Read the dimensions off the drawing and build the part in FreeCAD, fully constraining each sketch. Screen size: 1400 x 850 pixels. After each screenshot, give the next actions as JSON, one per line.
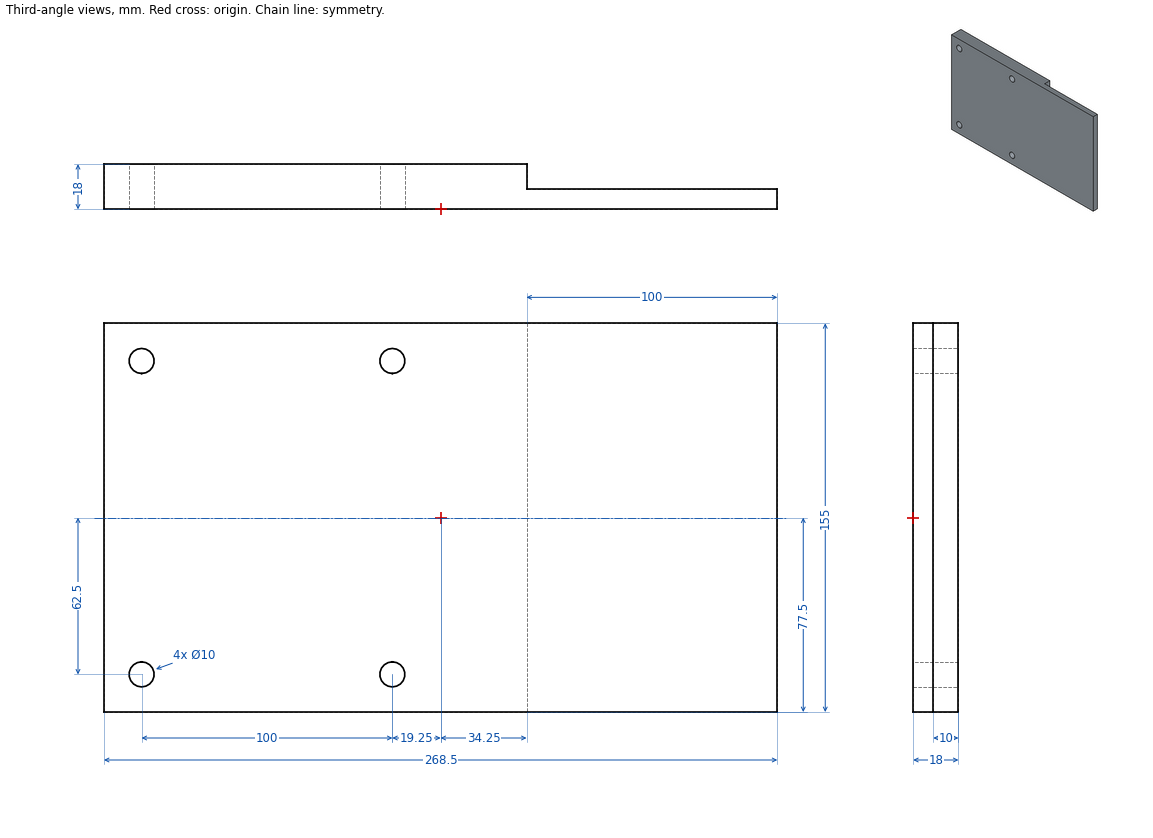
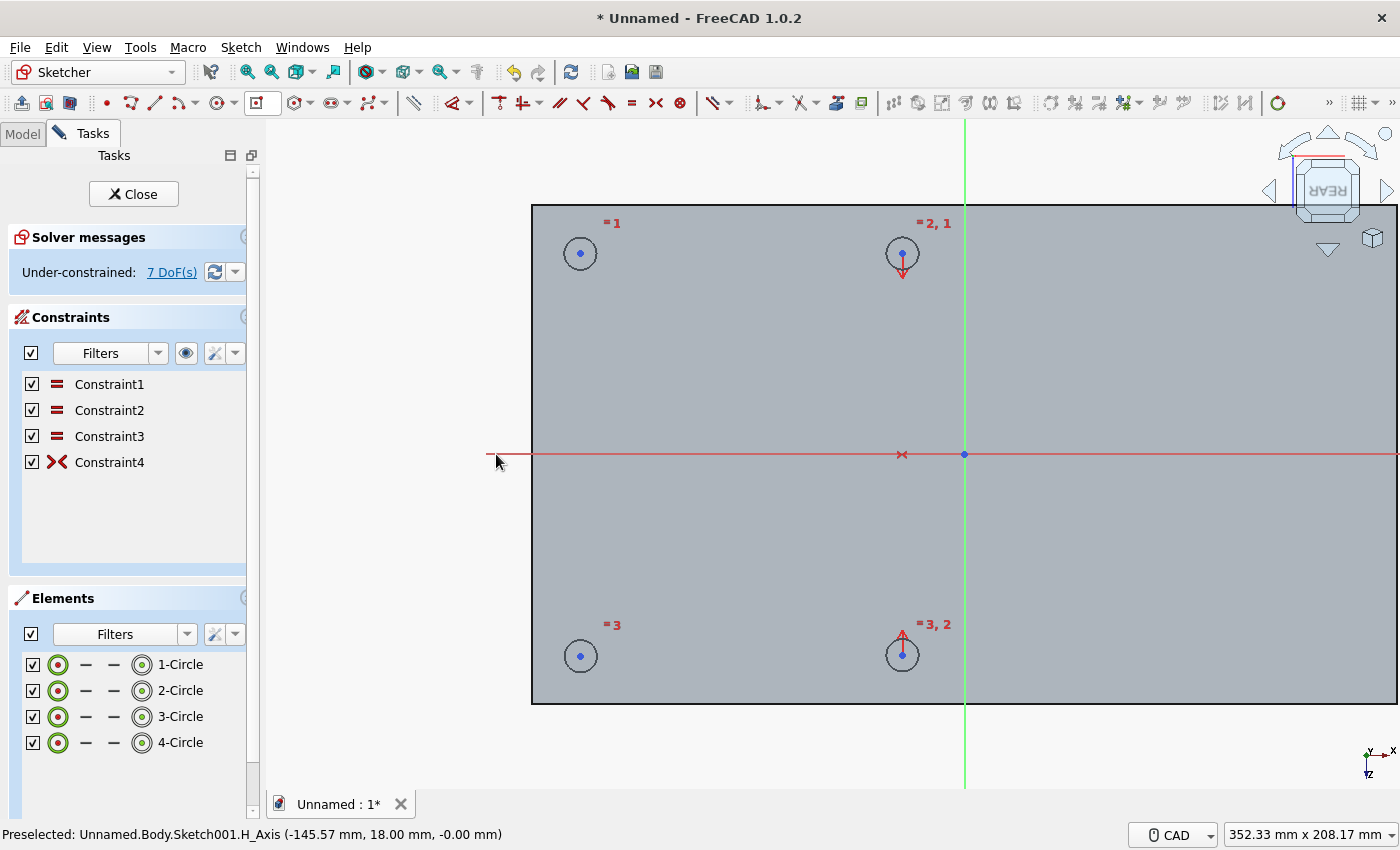
{"action": "left_click", "coordinate": [580, 254]}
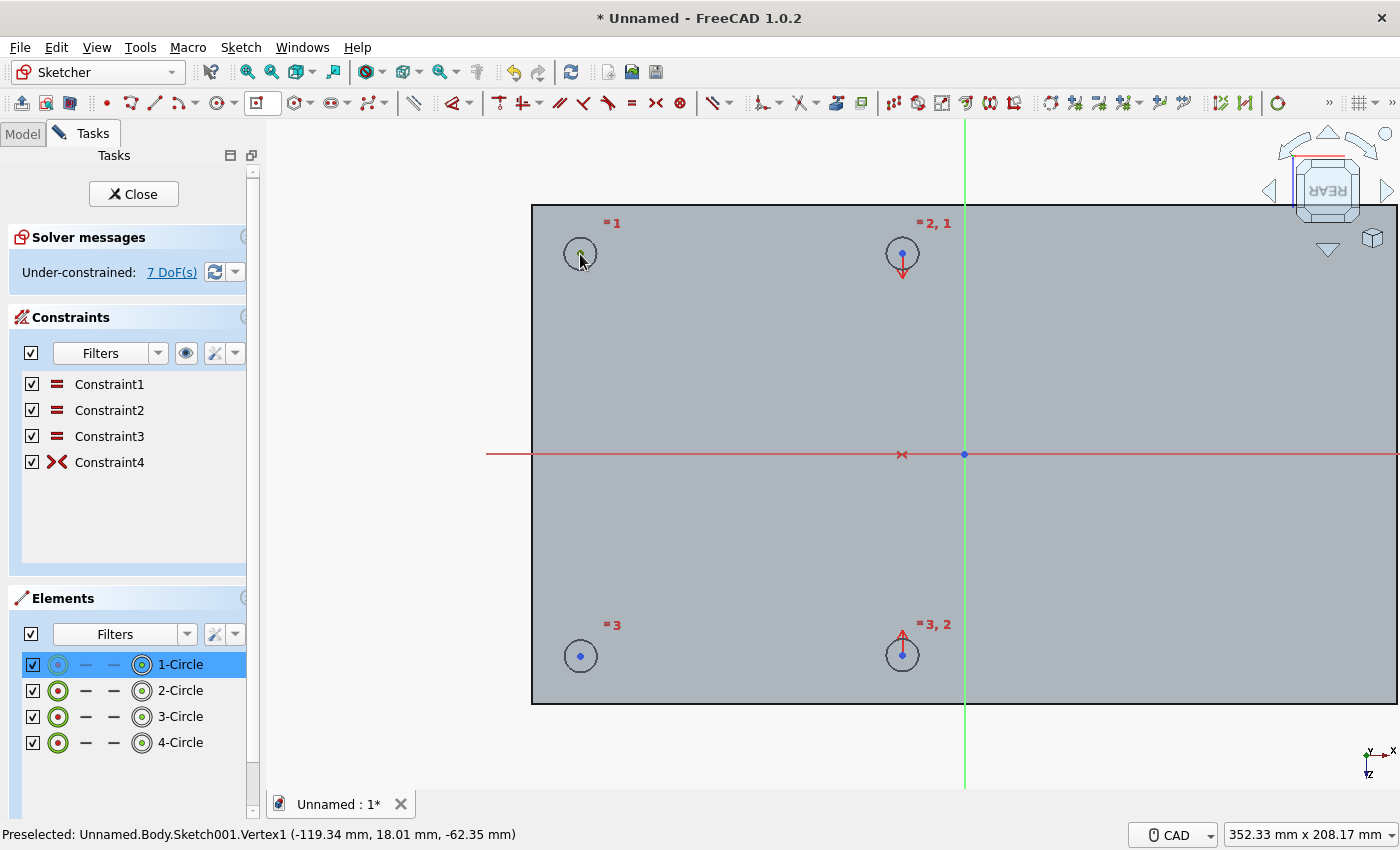
{"action": "left_click", "coordinate": [581, 656]}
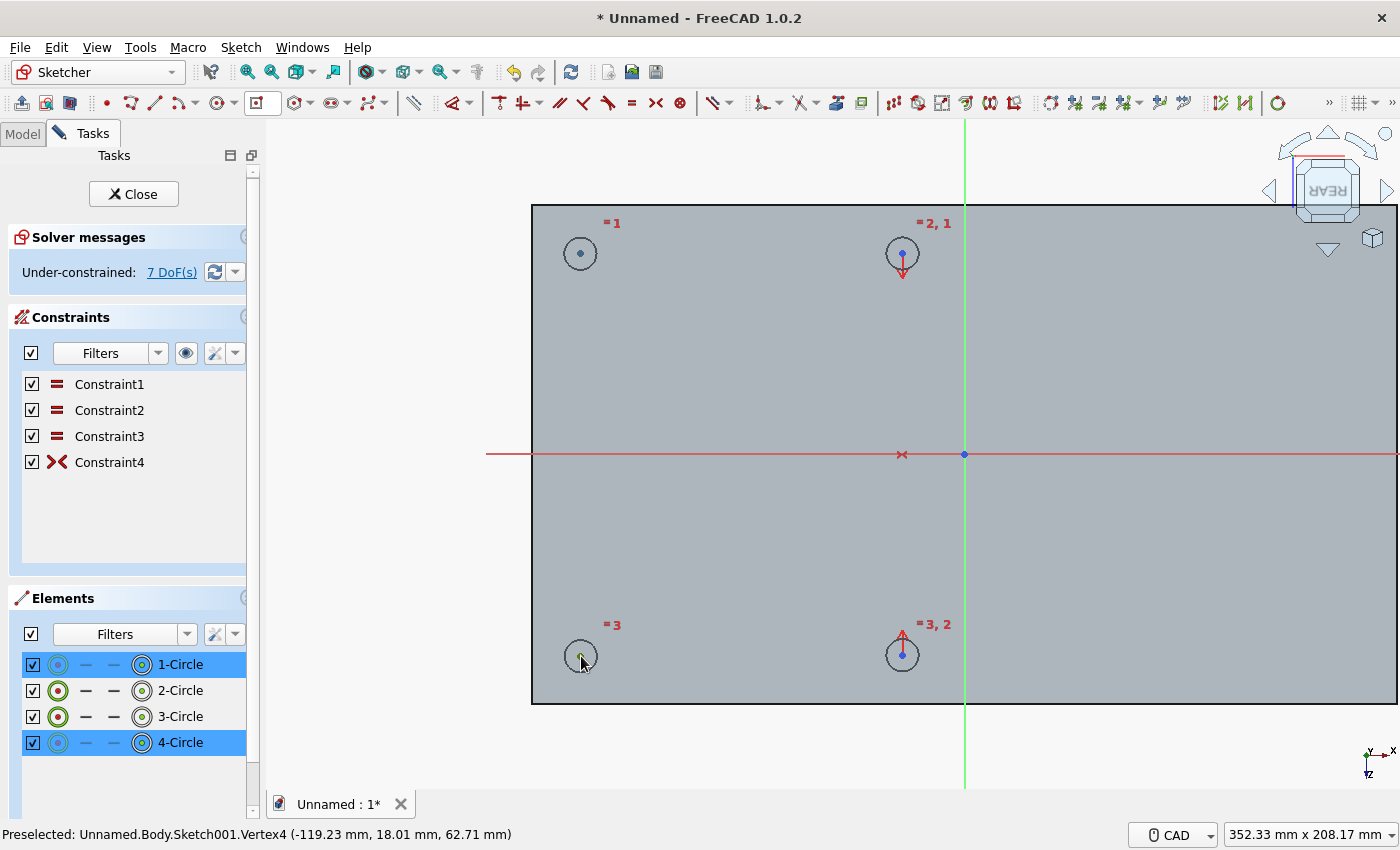
{"action": "left_click", "coordinate": [496, 454]}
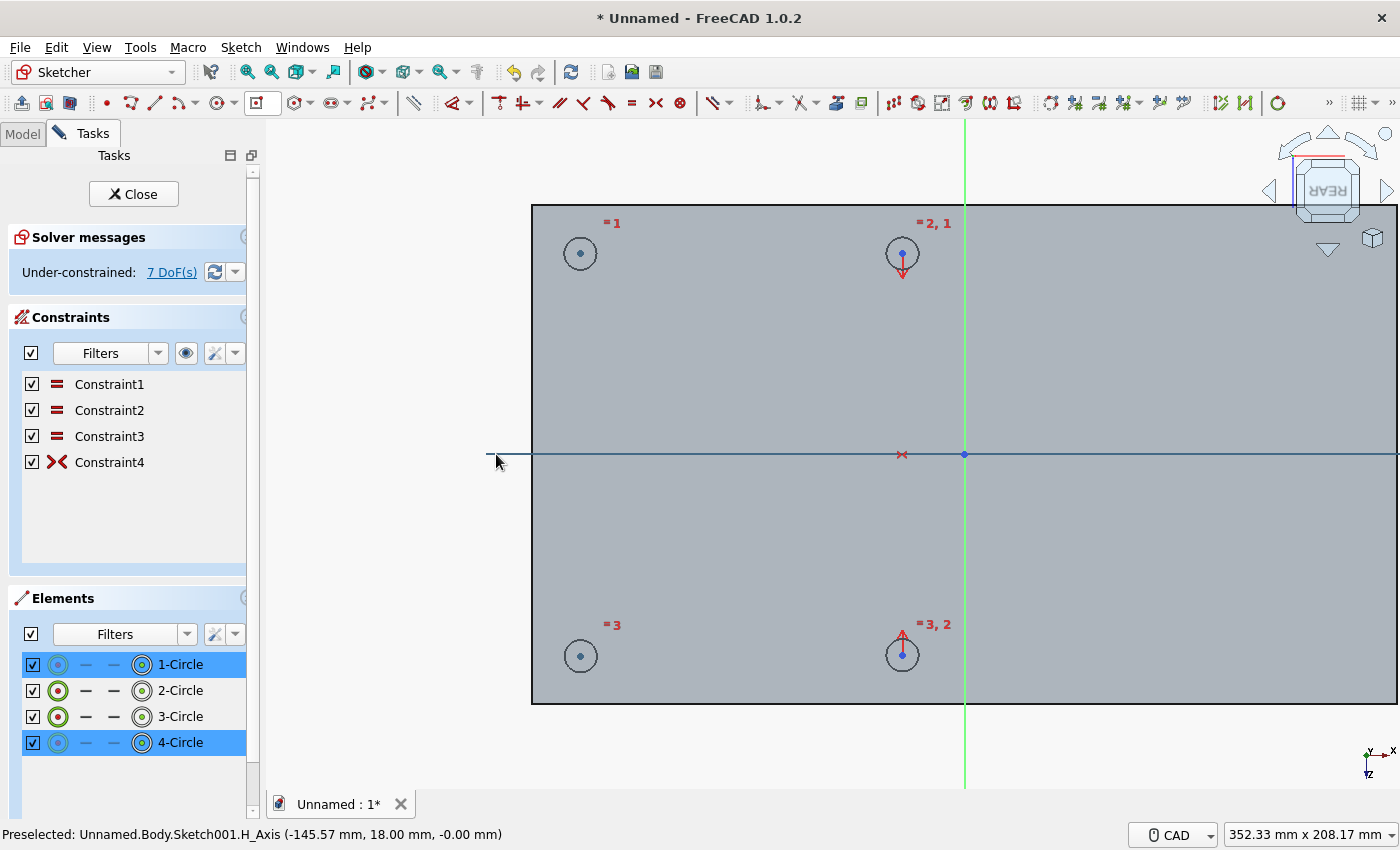
{"action": "left_click", "coordinate": [656, 104]}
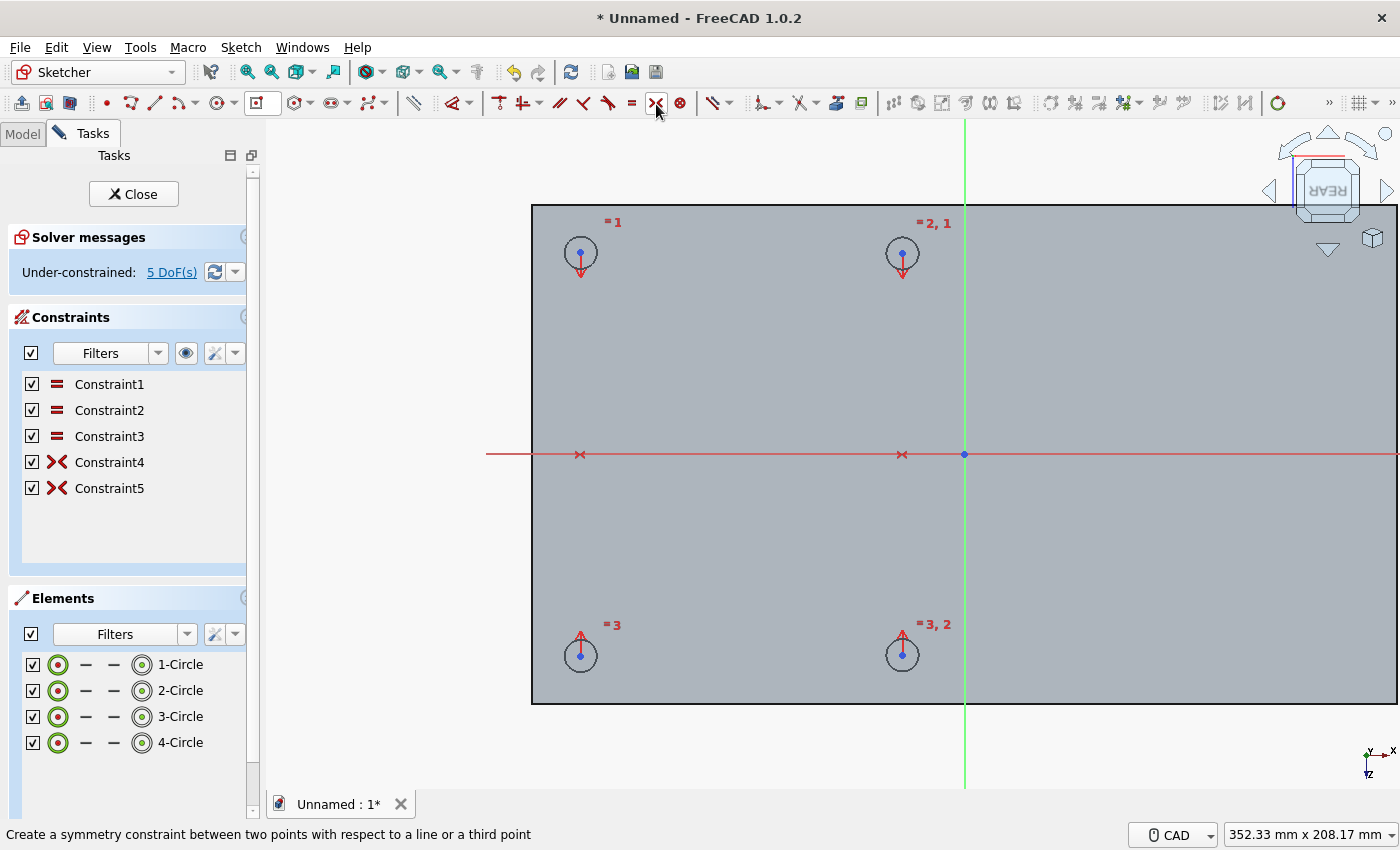
{"action": "left_click", "coordinate": [452, 104]}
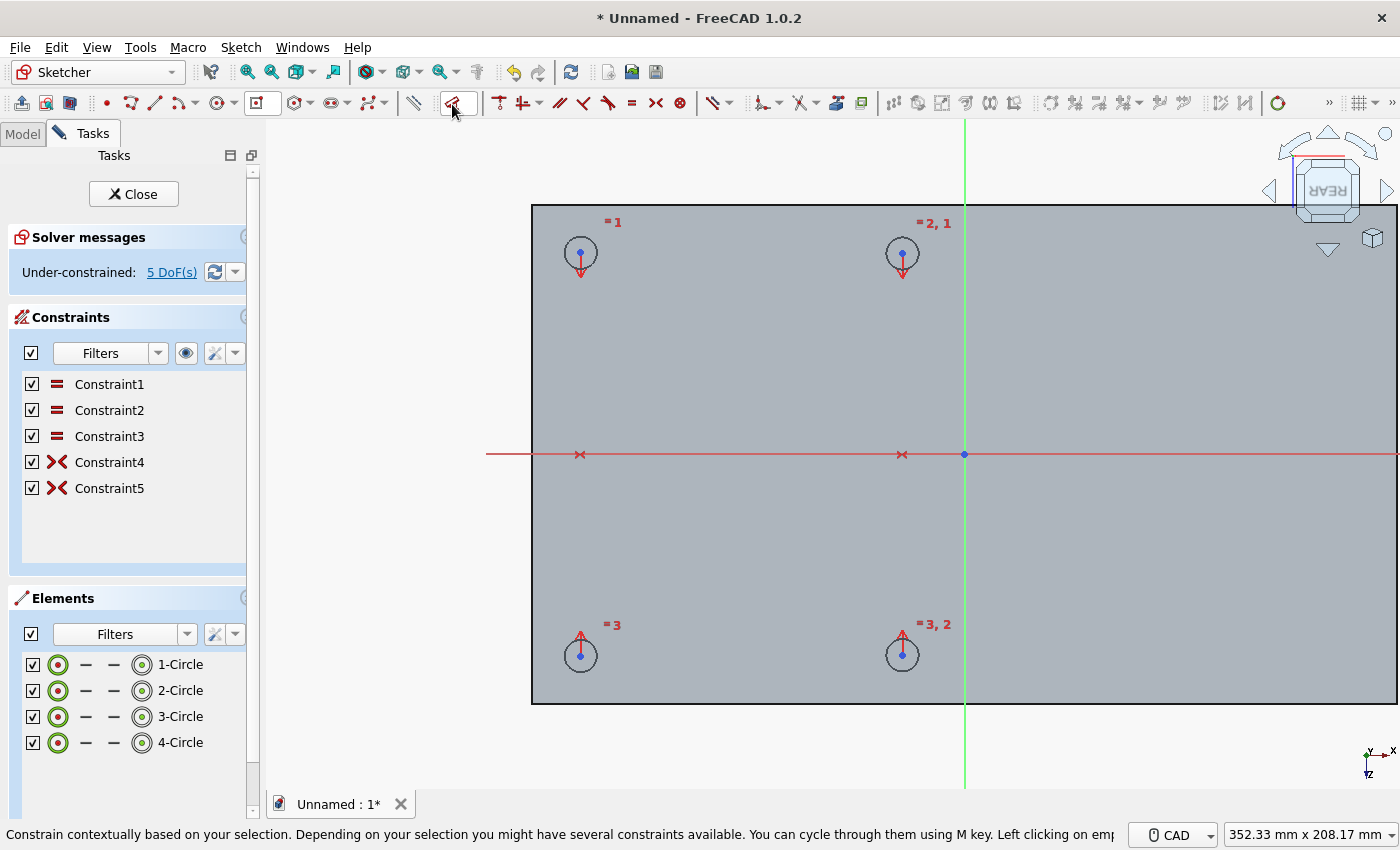
{"action": "scroll", "coordinate": [592, 241], "scroll_direction": "up", "scroll_amount": 2}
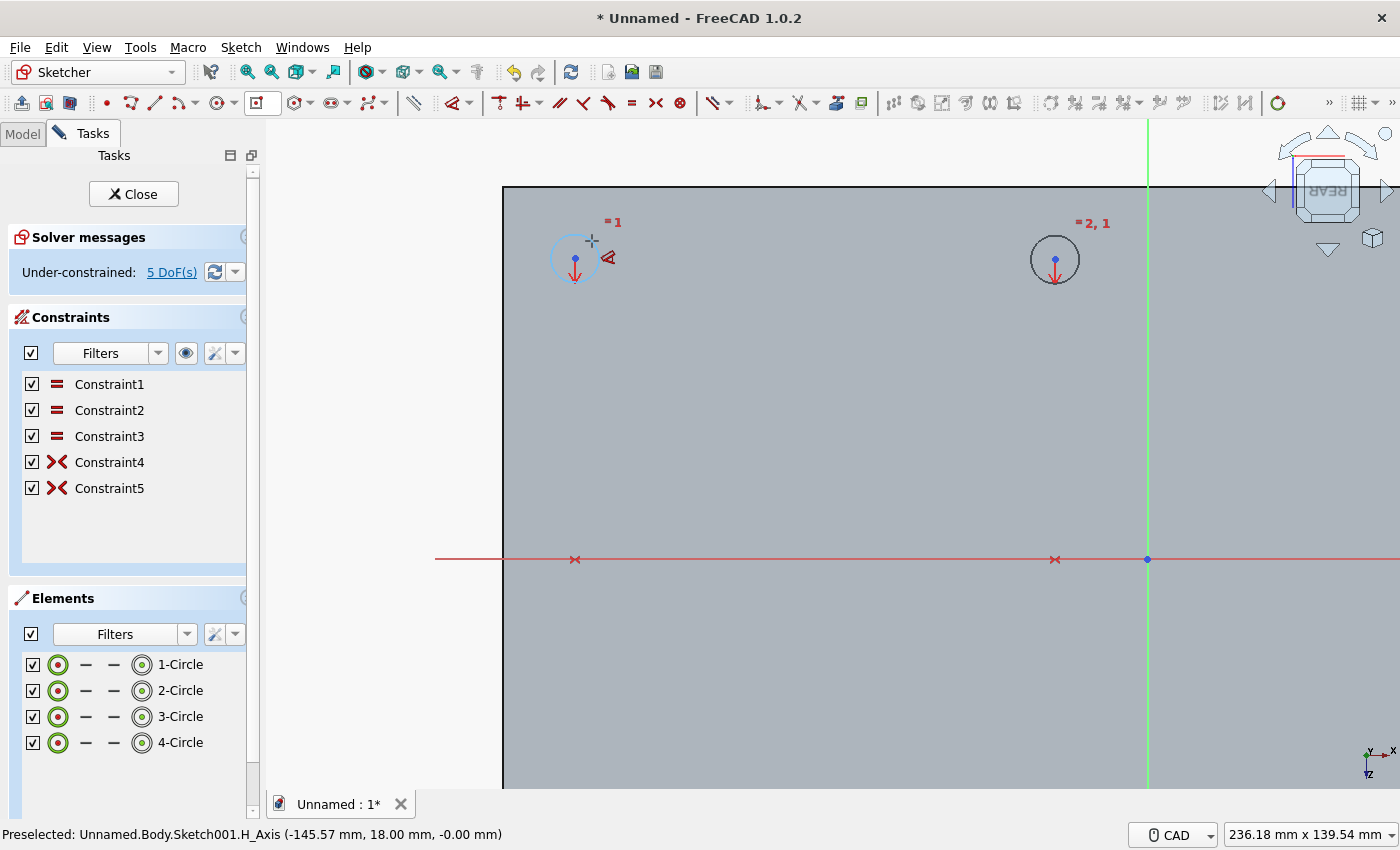
{"action": "left_click", "coordinate": [592, 241]}
{"action": "left_click", "coordinate": [614, 218]}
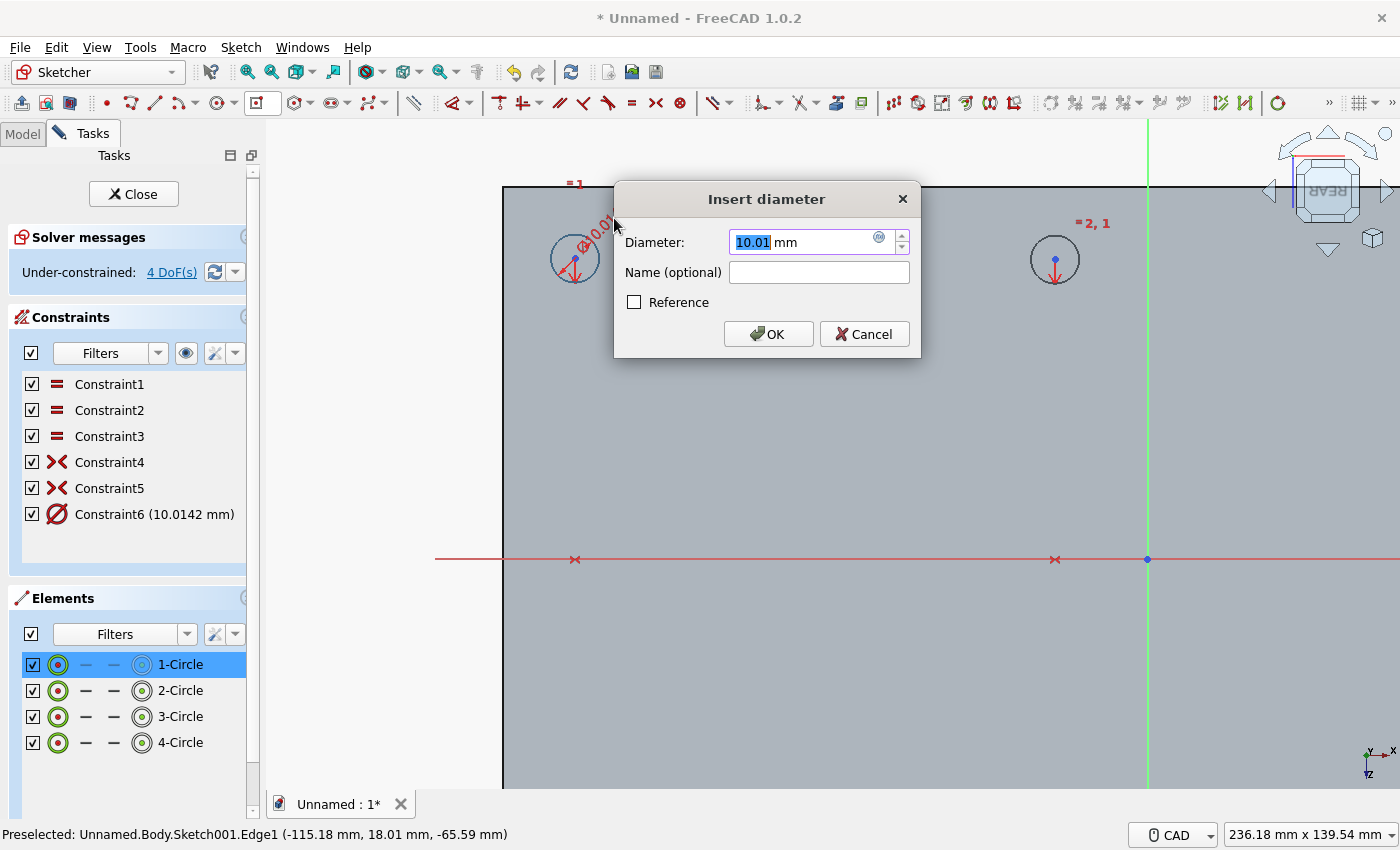
{"action": "type", "text": "10"}
{"action": "key", "text": "Return"}